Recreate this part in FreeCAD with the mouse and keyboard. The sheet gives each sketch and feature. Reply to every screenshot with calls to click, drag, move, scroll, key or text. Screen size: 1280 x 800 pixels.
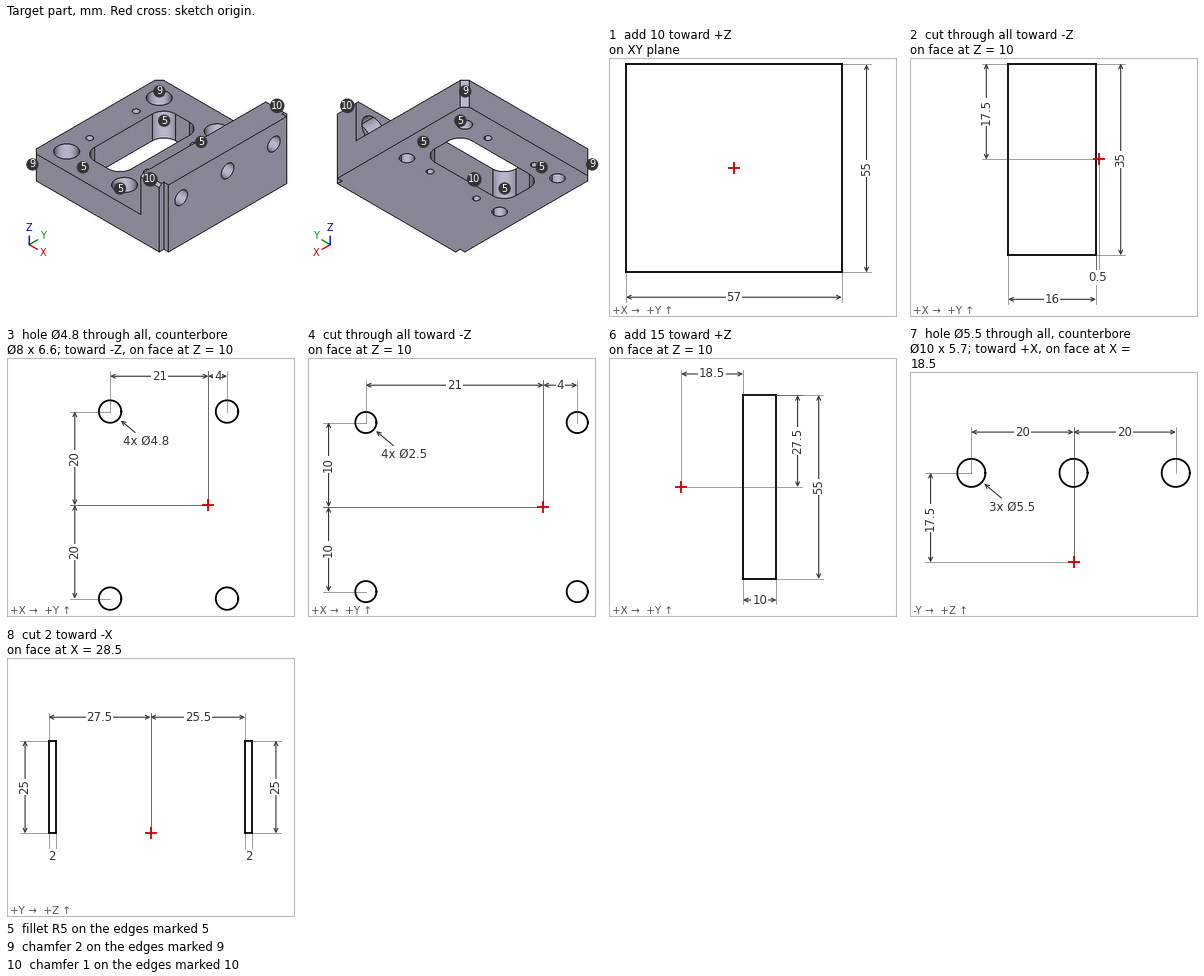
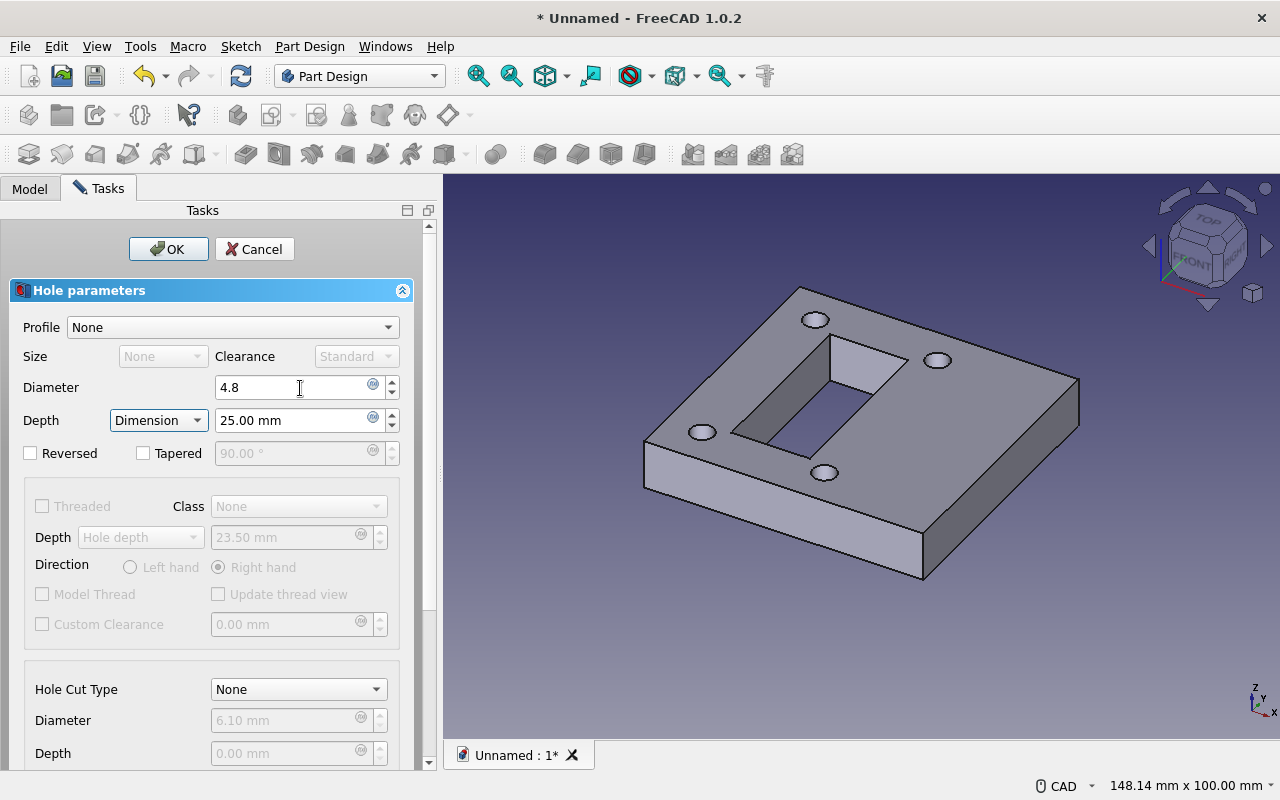
click(160, 420)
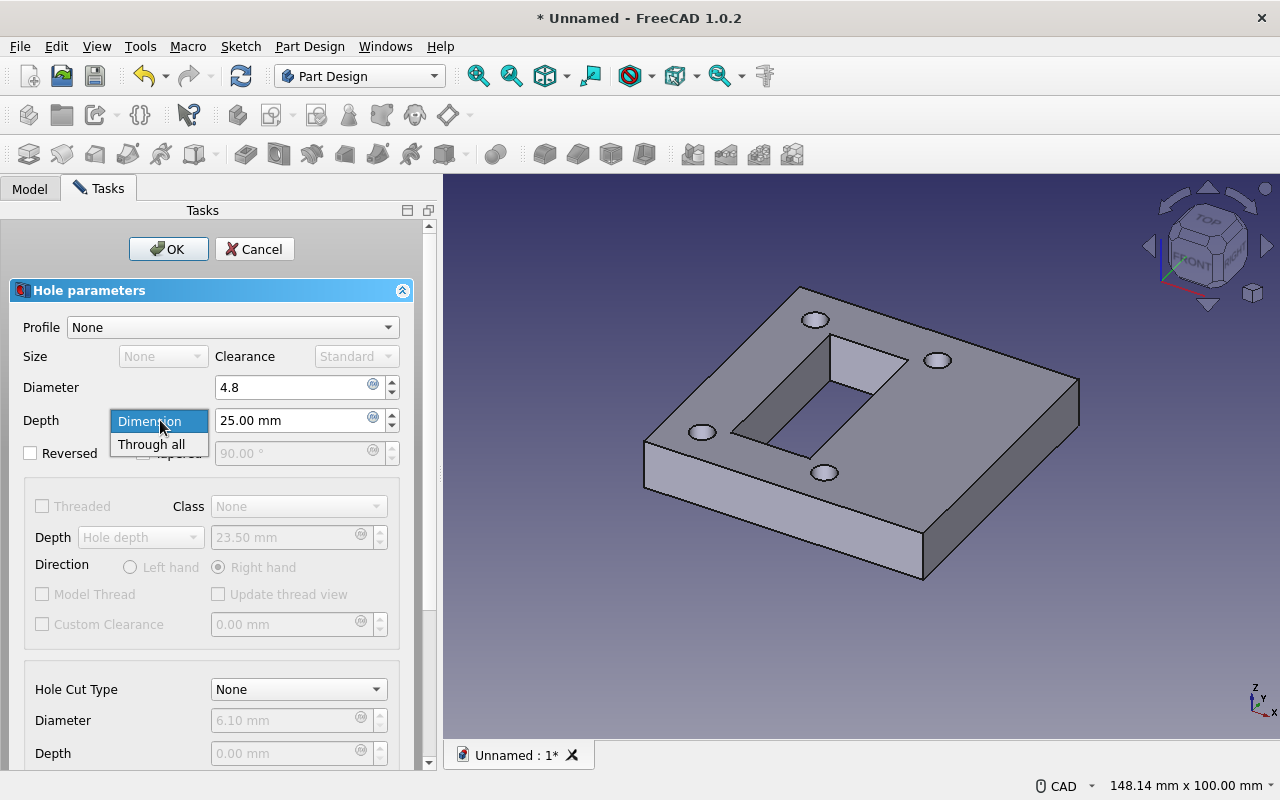
click(158, 444)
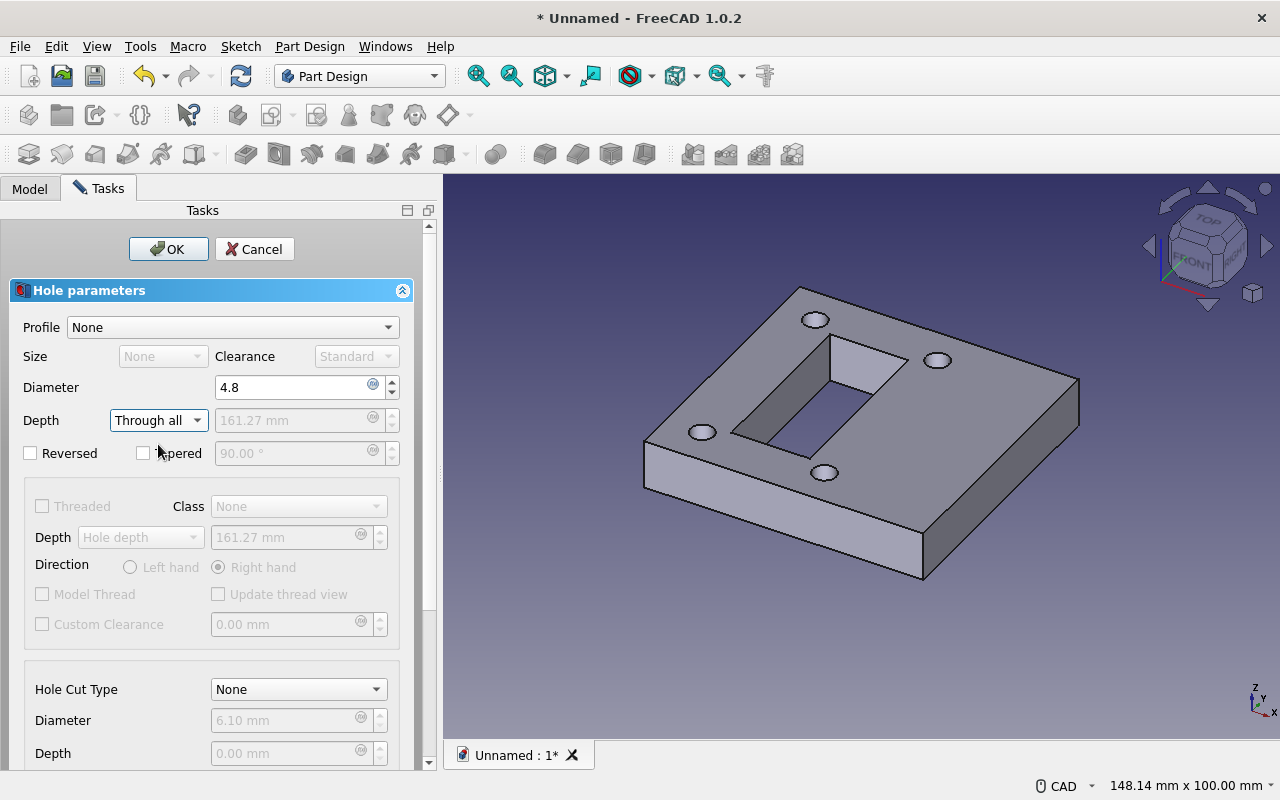
click(300, 690)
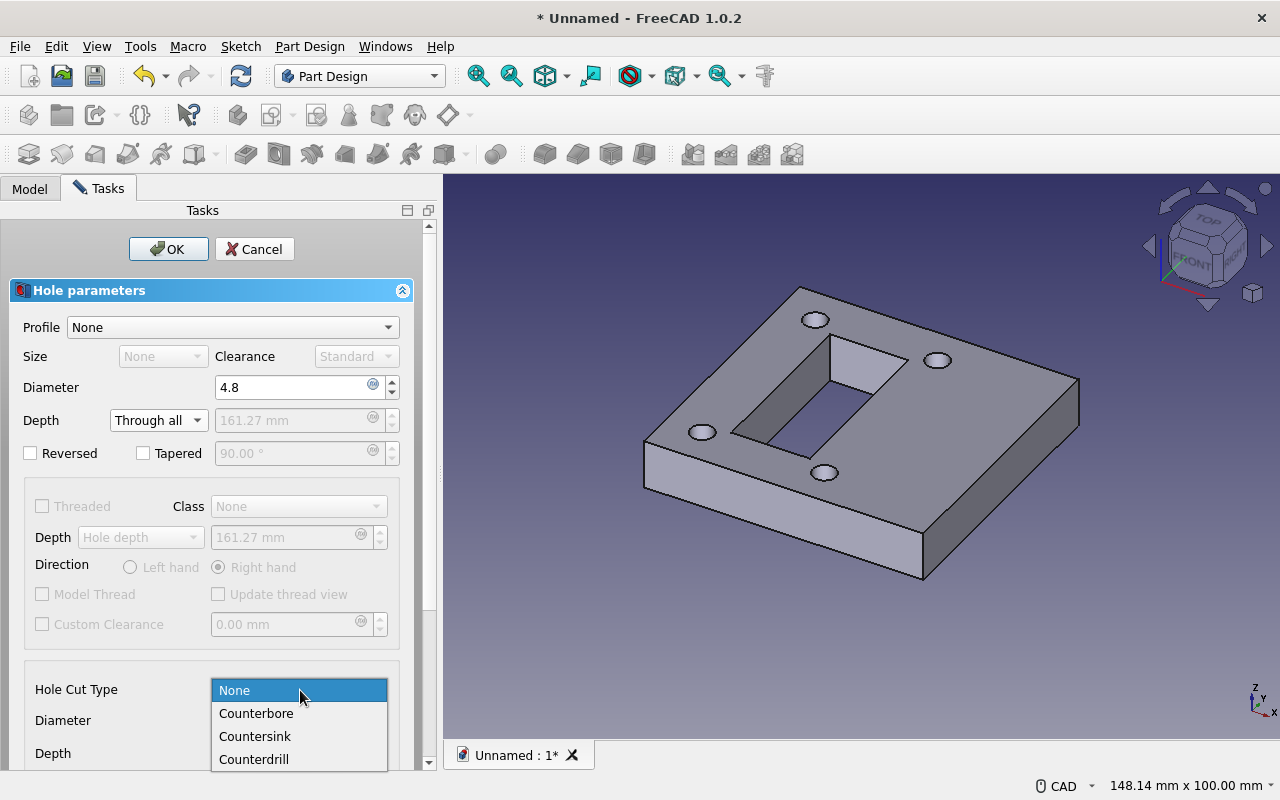
click(298, 714)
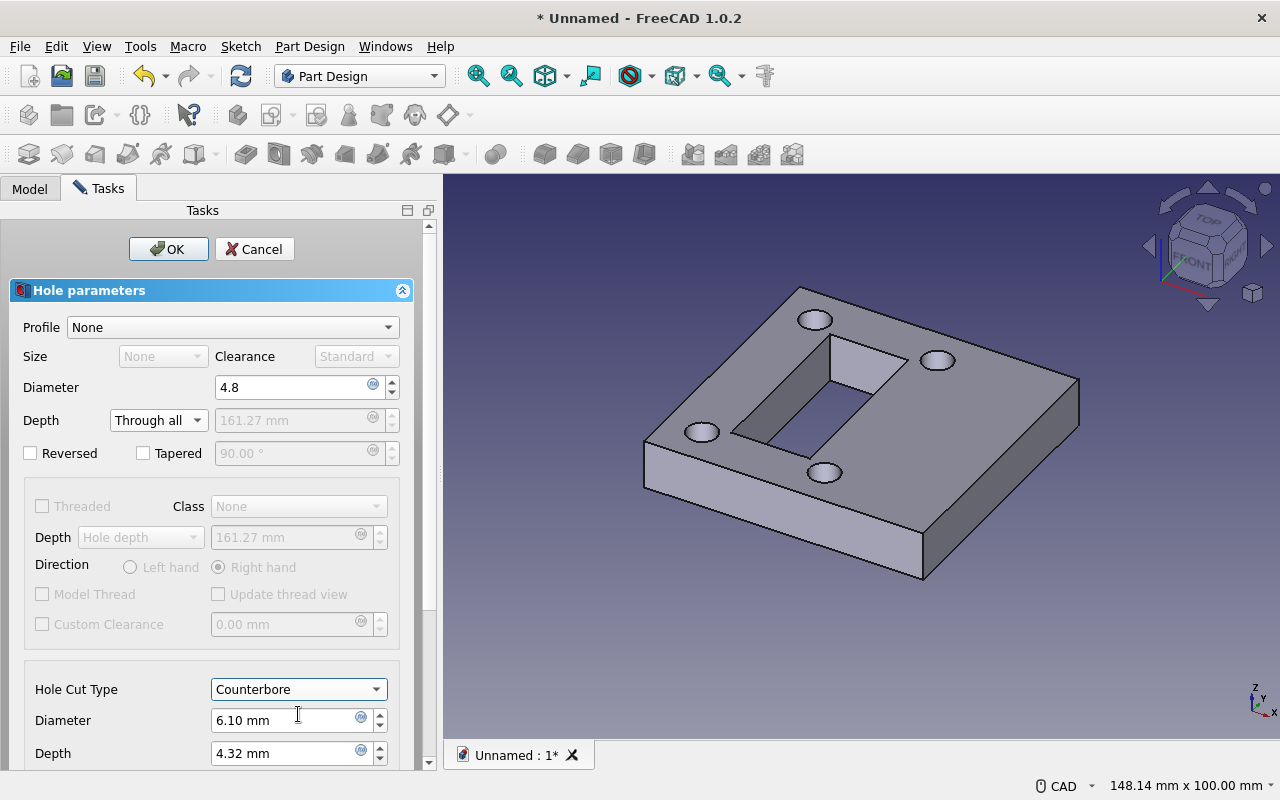
triple_click(292, 720)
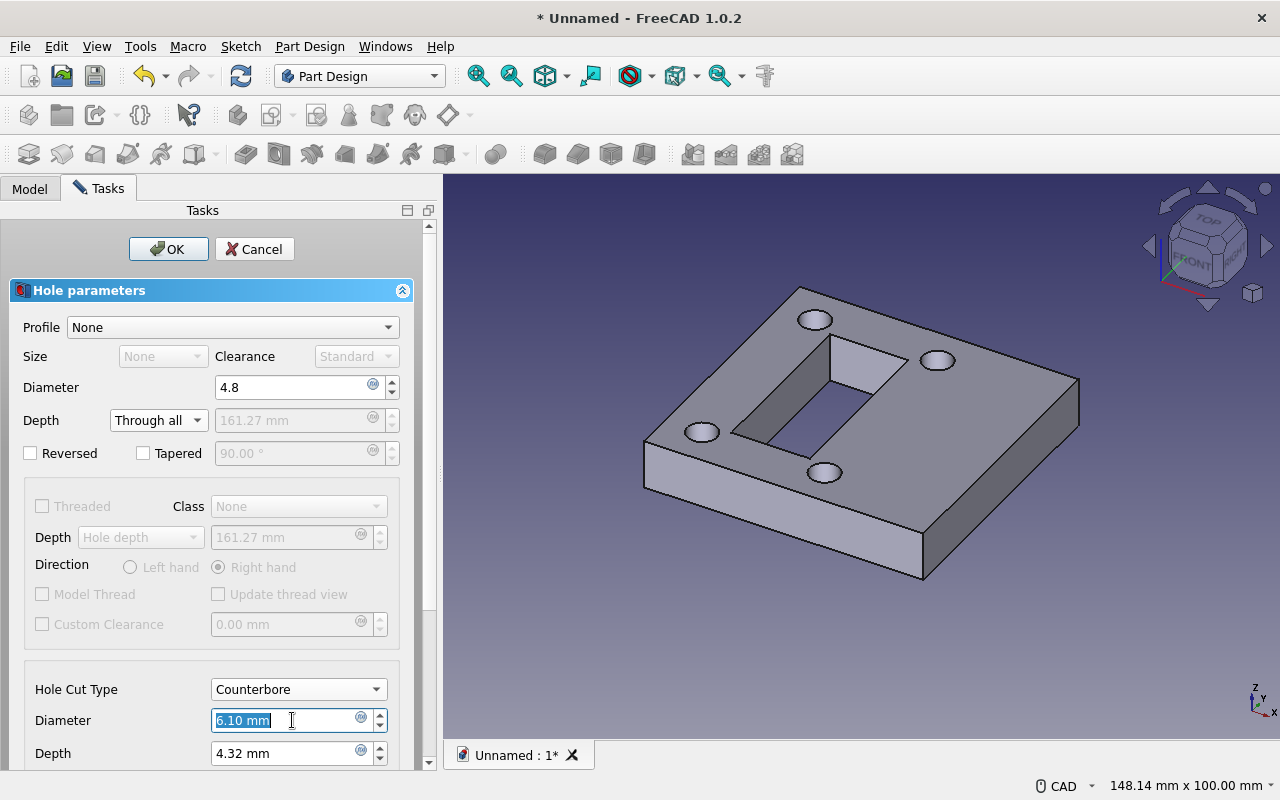
text(8)
key(Tab)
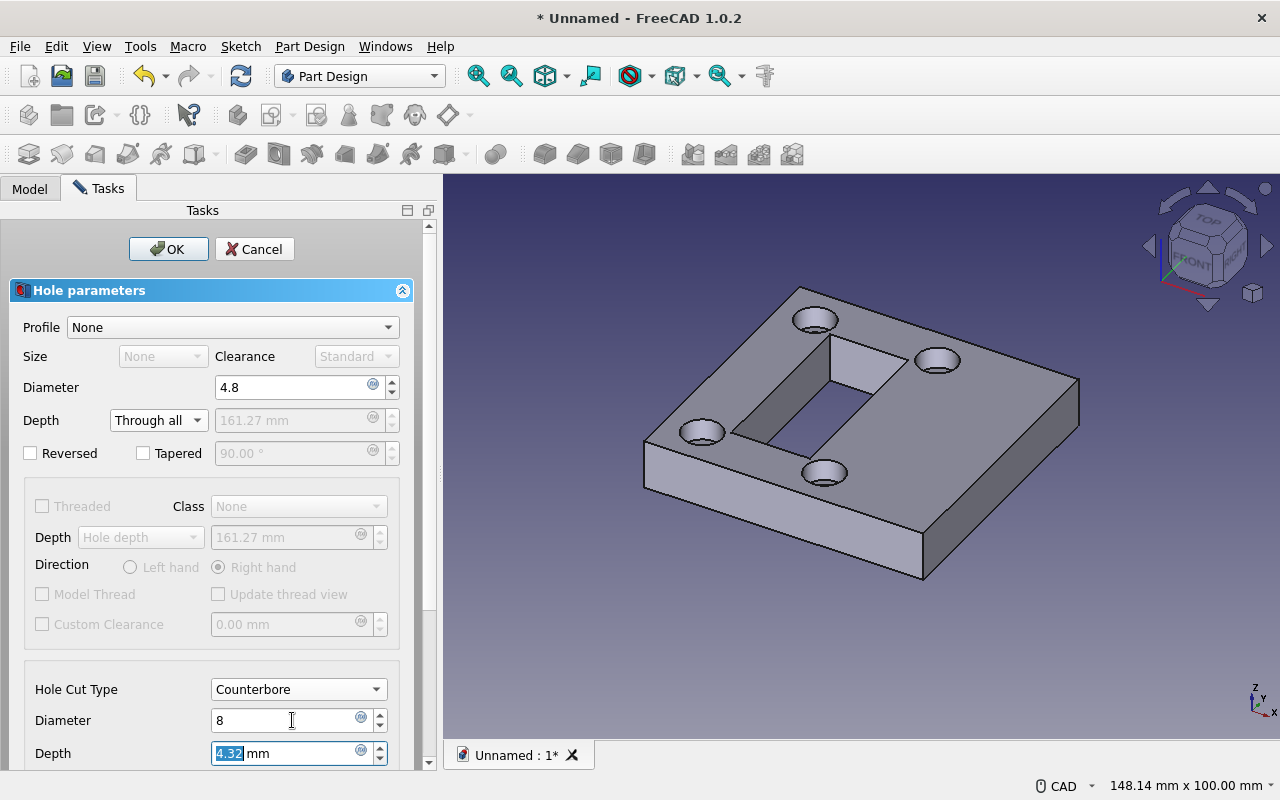
text(6.6)
key(Tab)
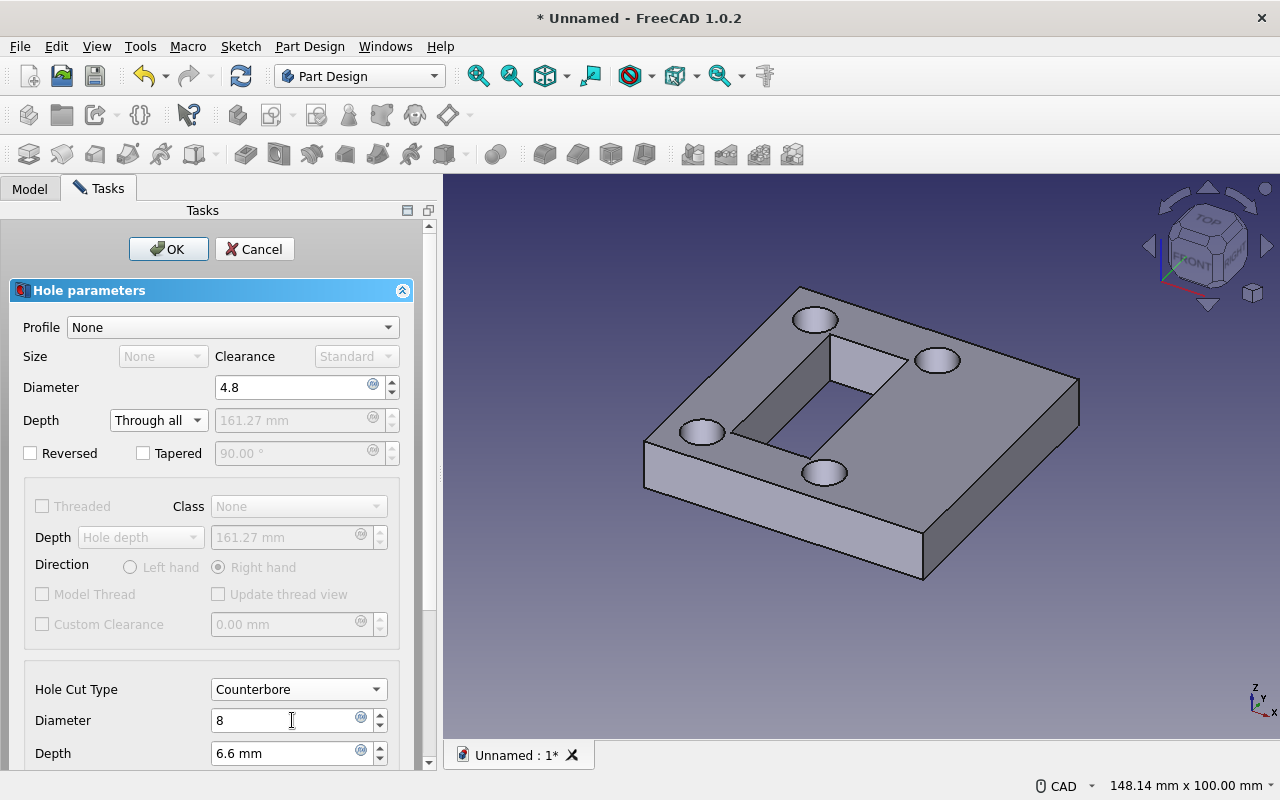
click(169, 249)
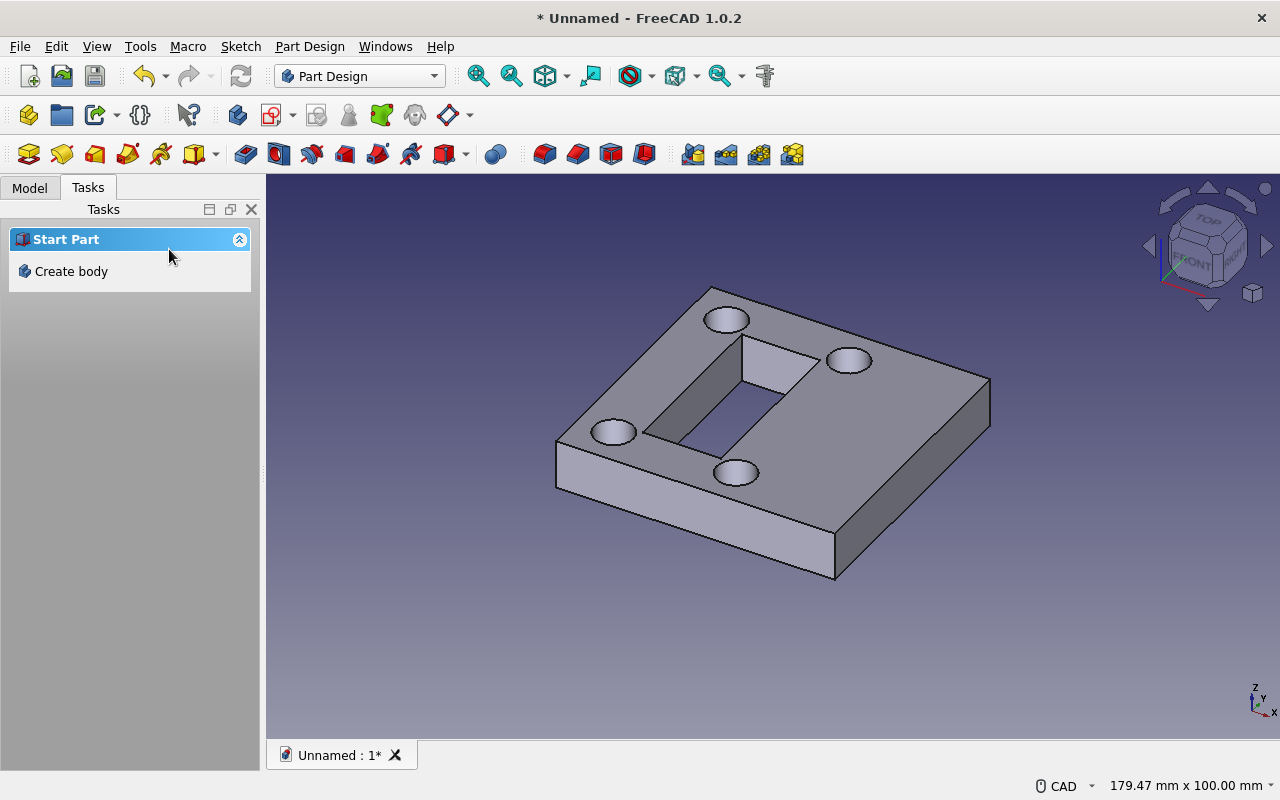
click(875, 414)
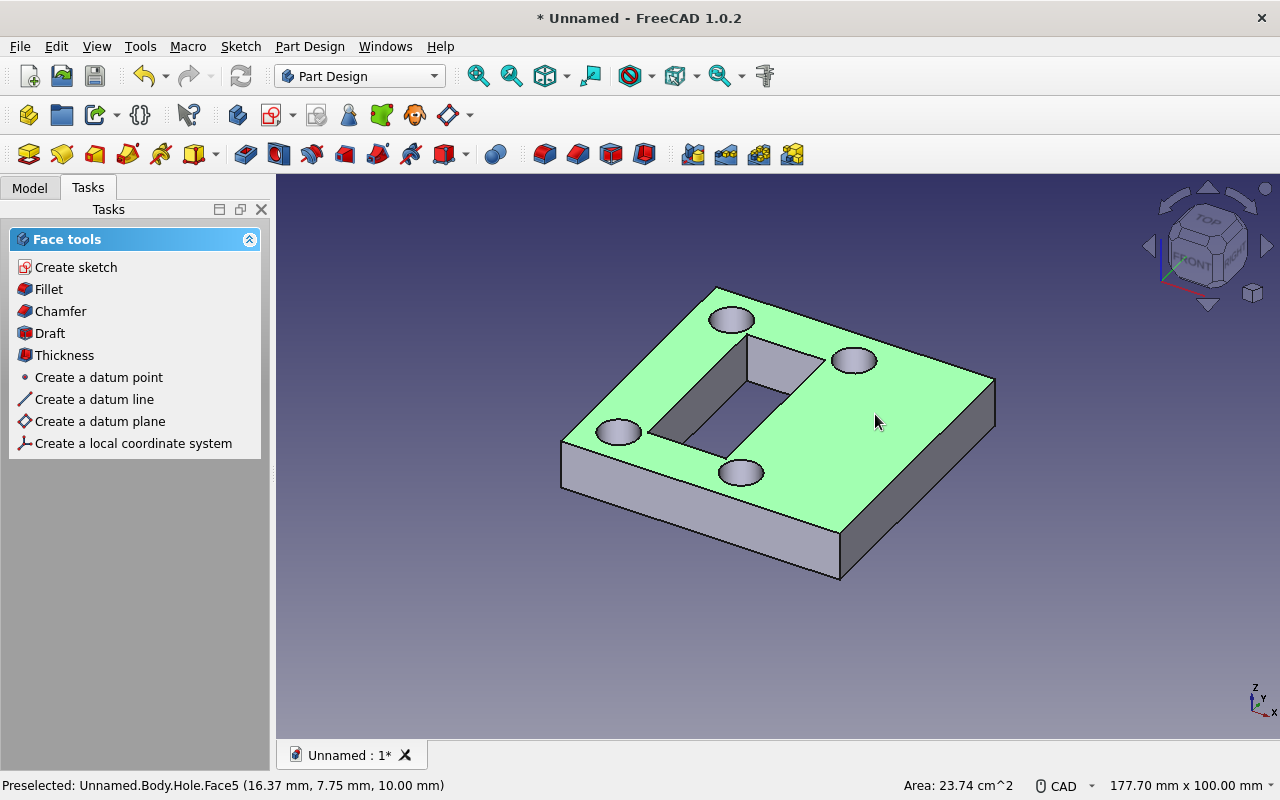
click(270, 116)